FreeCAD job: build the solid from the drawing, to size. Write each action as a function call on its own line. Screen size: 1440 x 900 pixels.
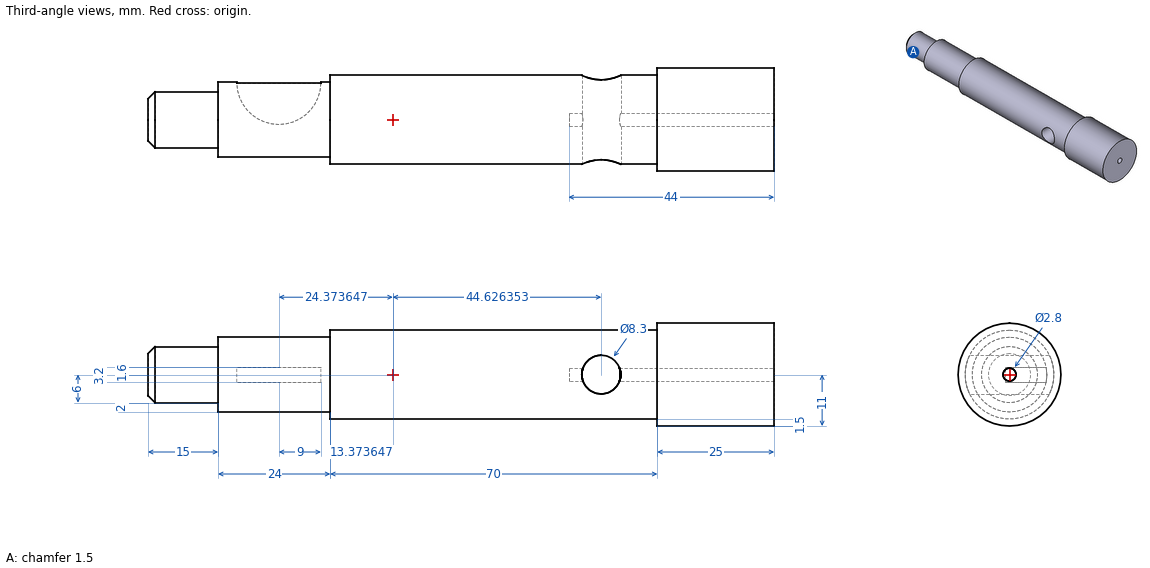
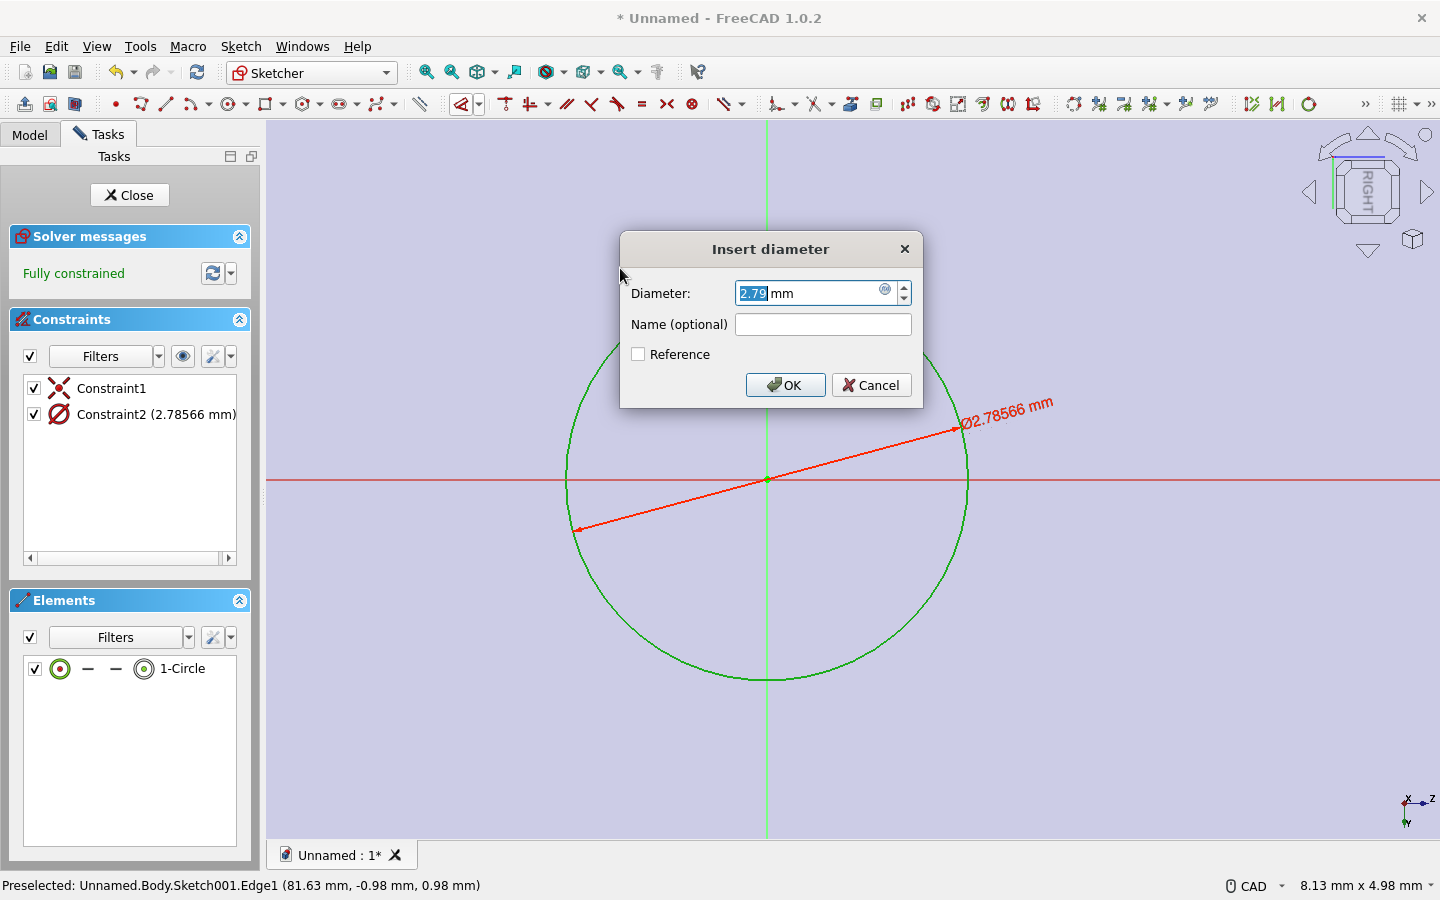
text(2.8)
key(Return)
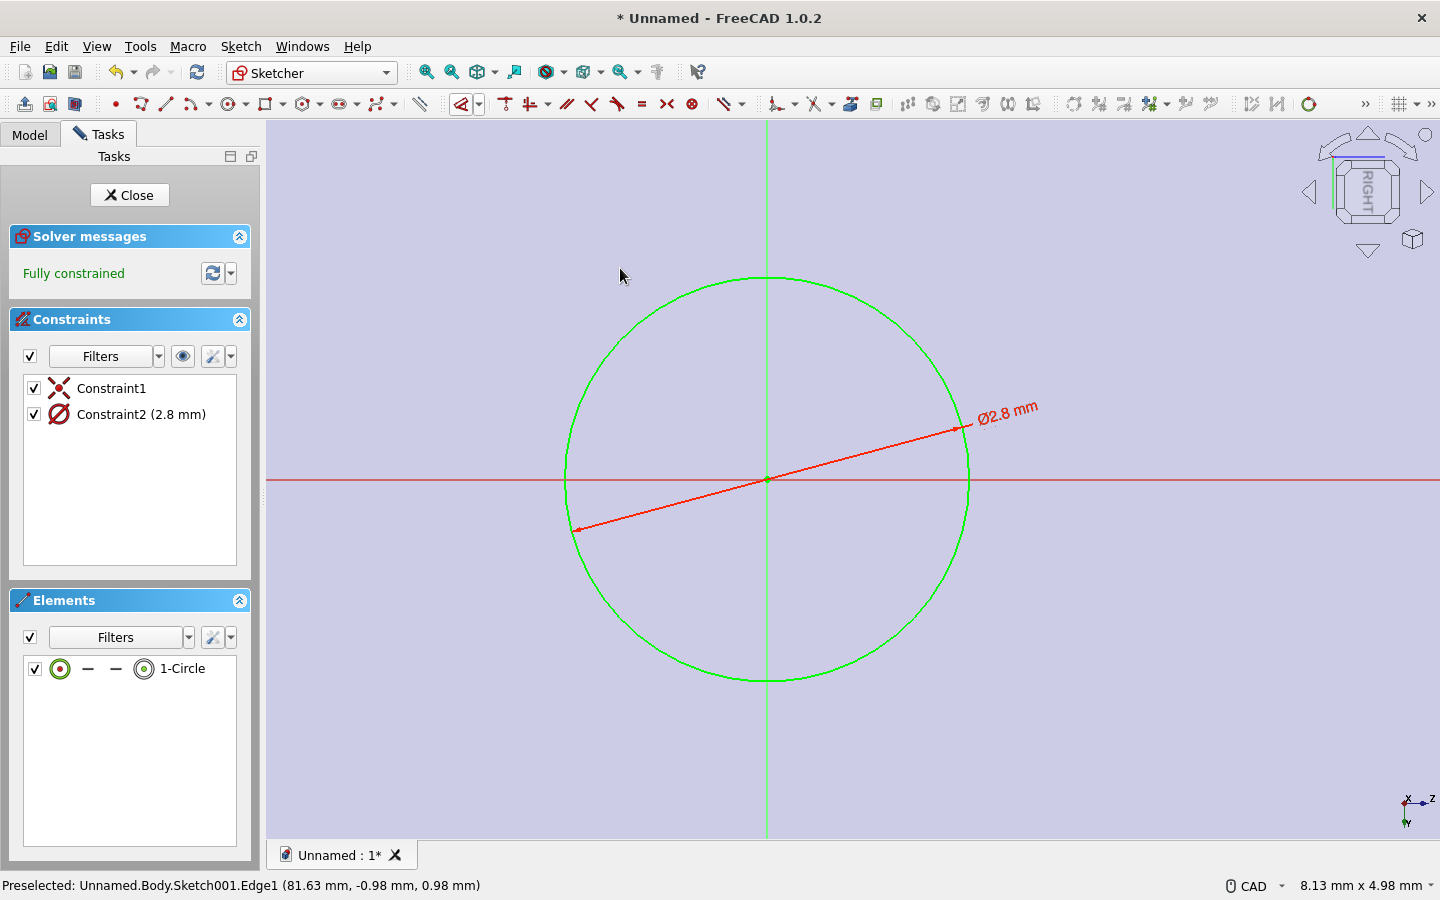
click(130, 195)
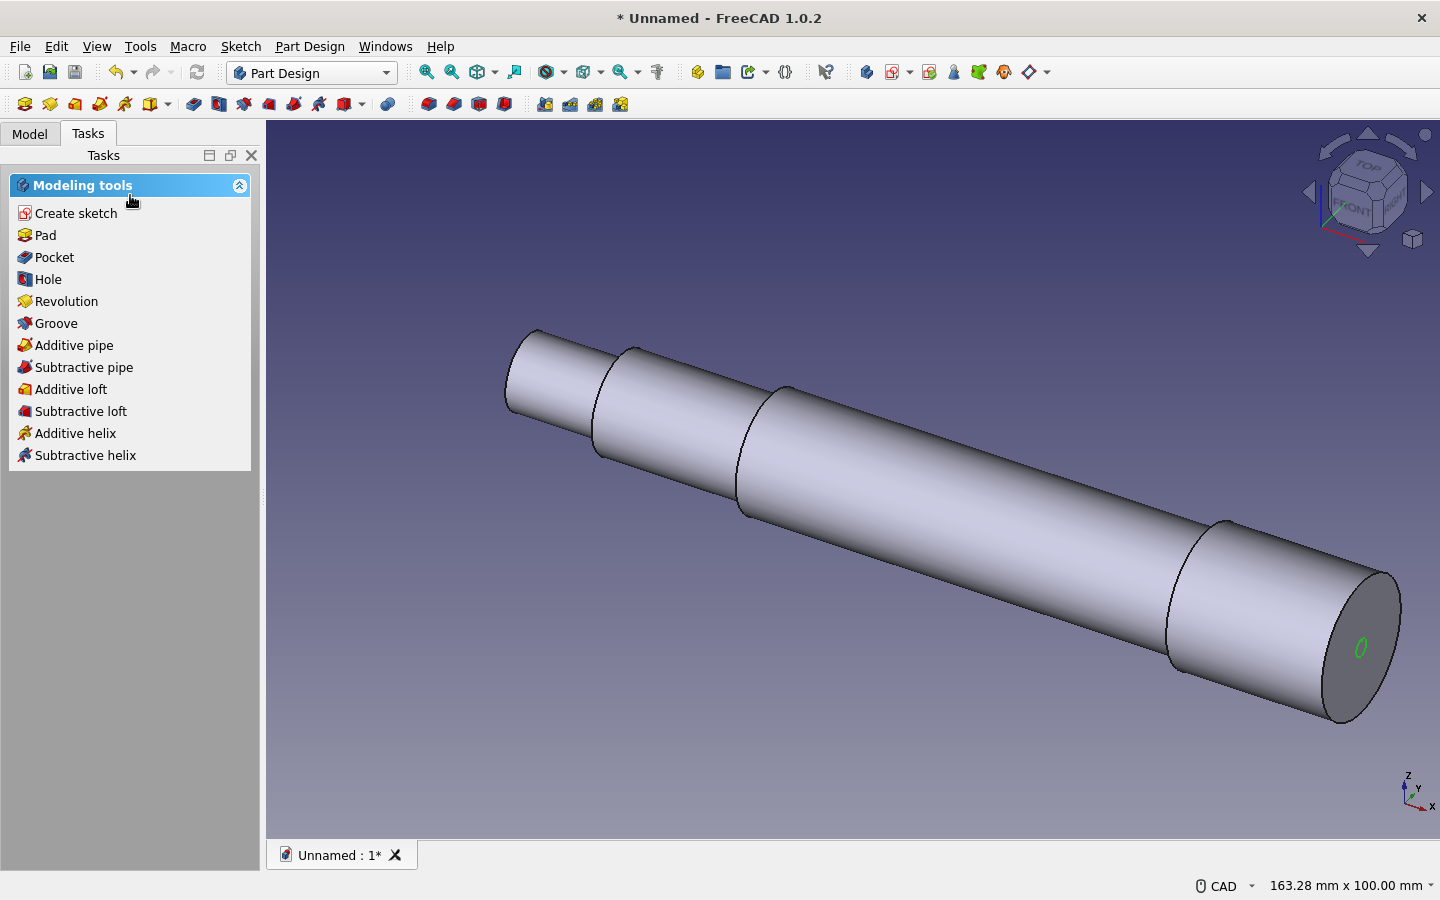
click(194, 104)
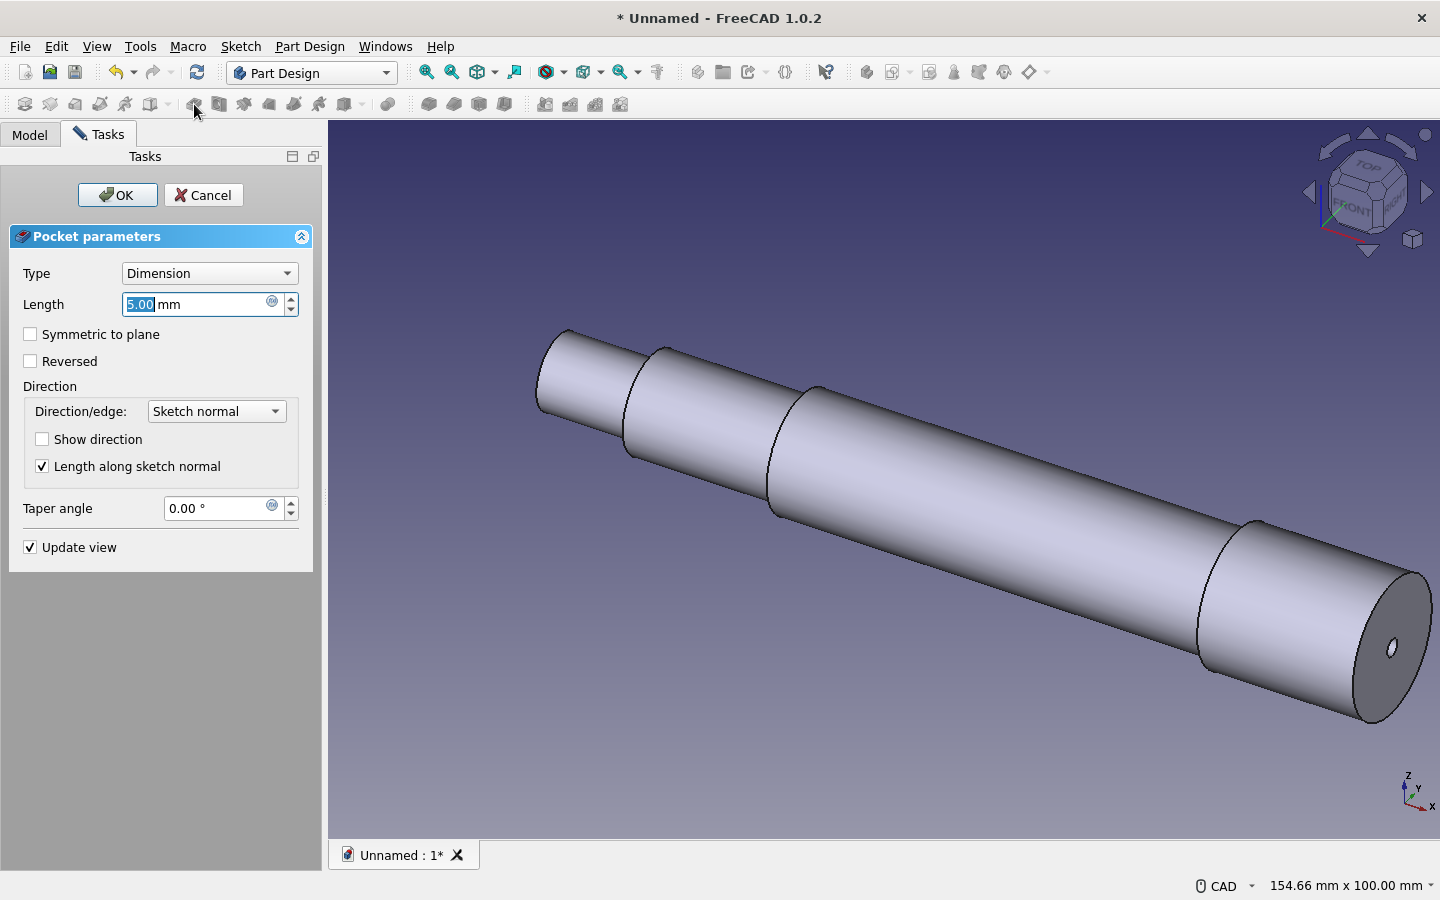
text(44)
key(Tab)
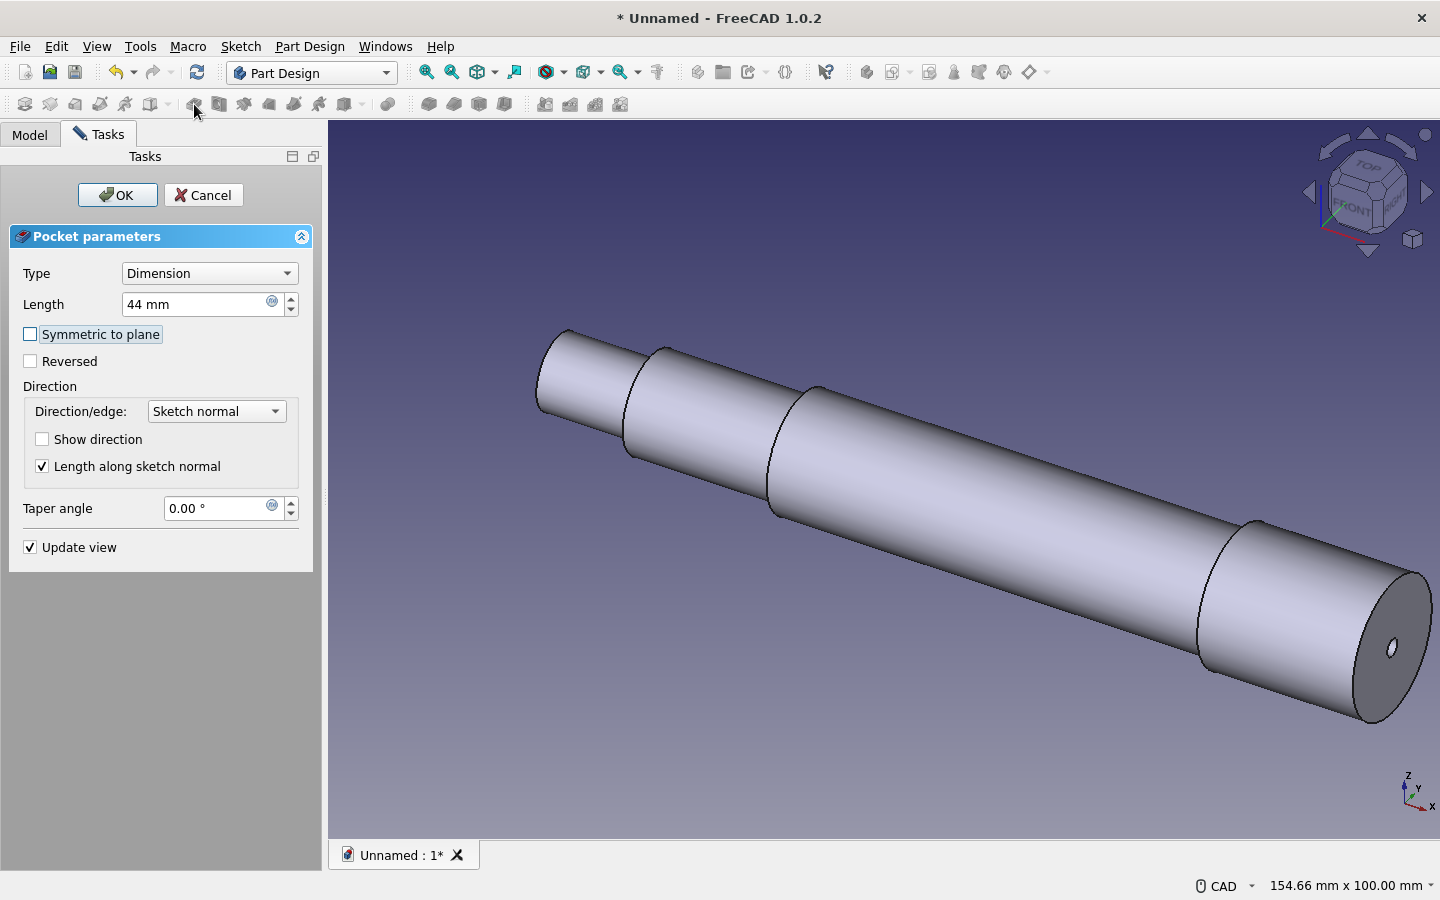
click(118, 195)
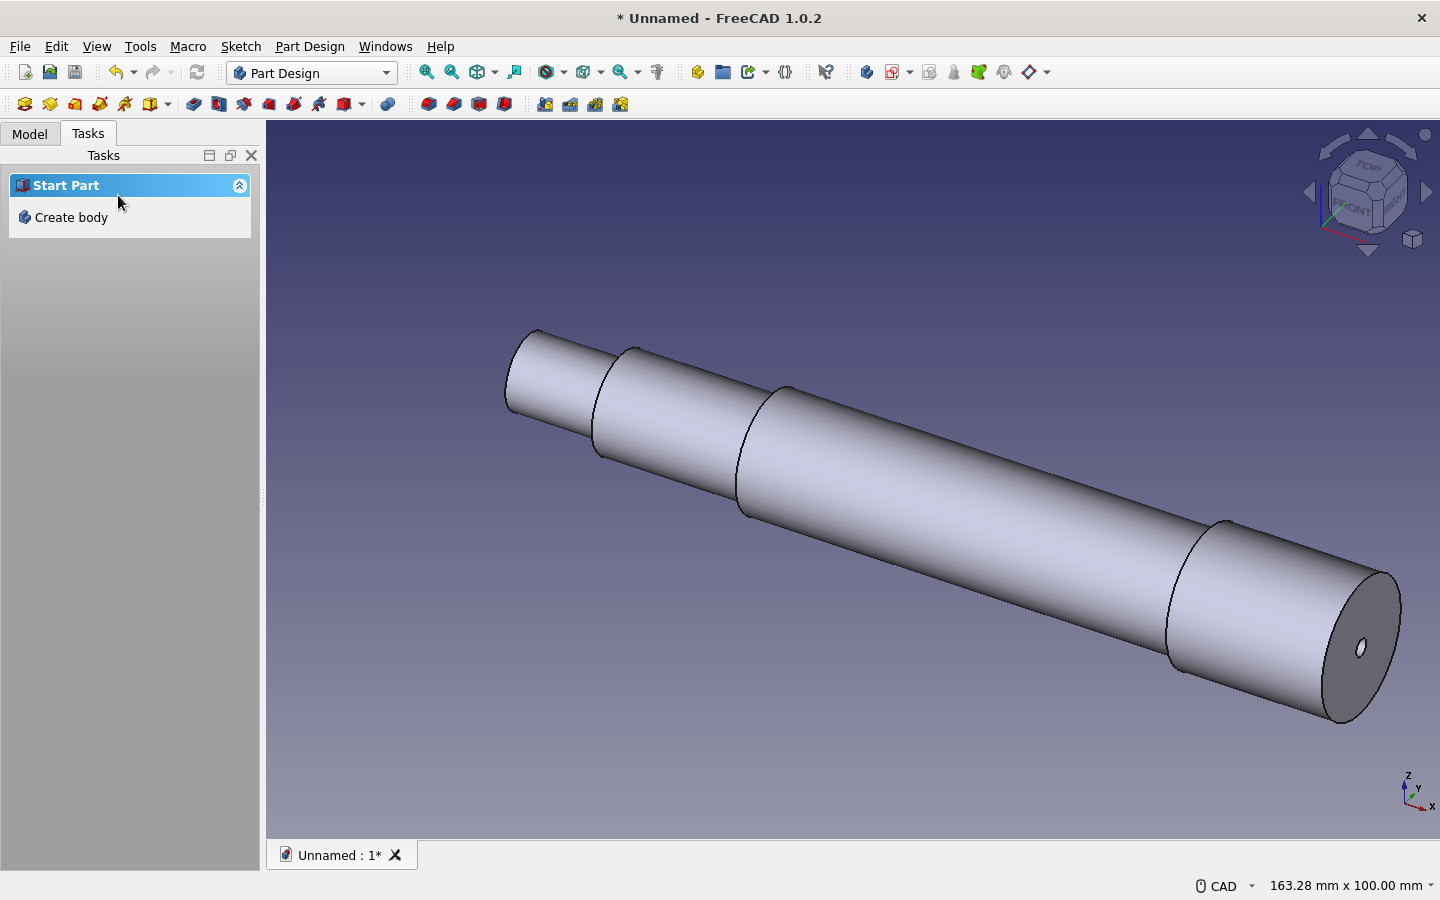
click(892, 72)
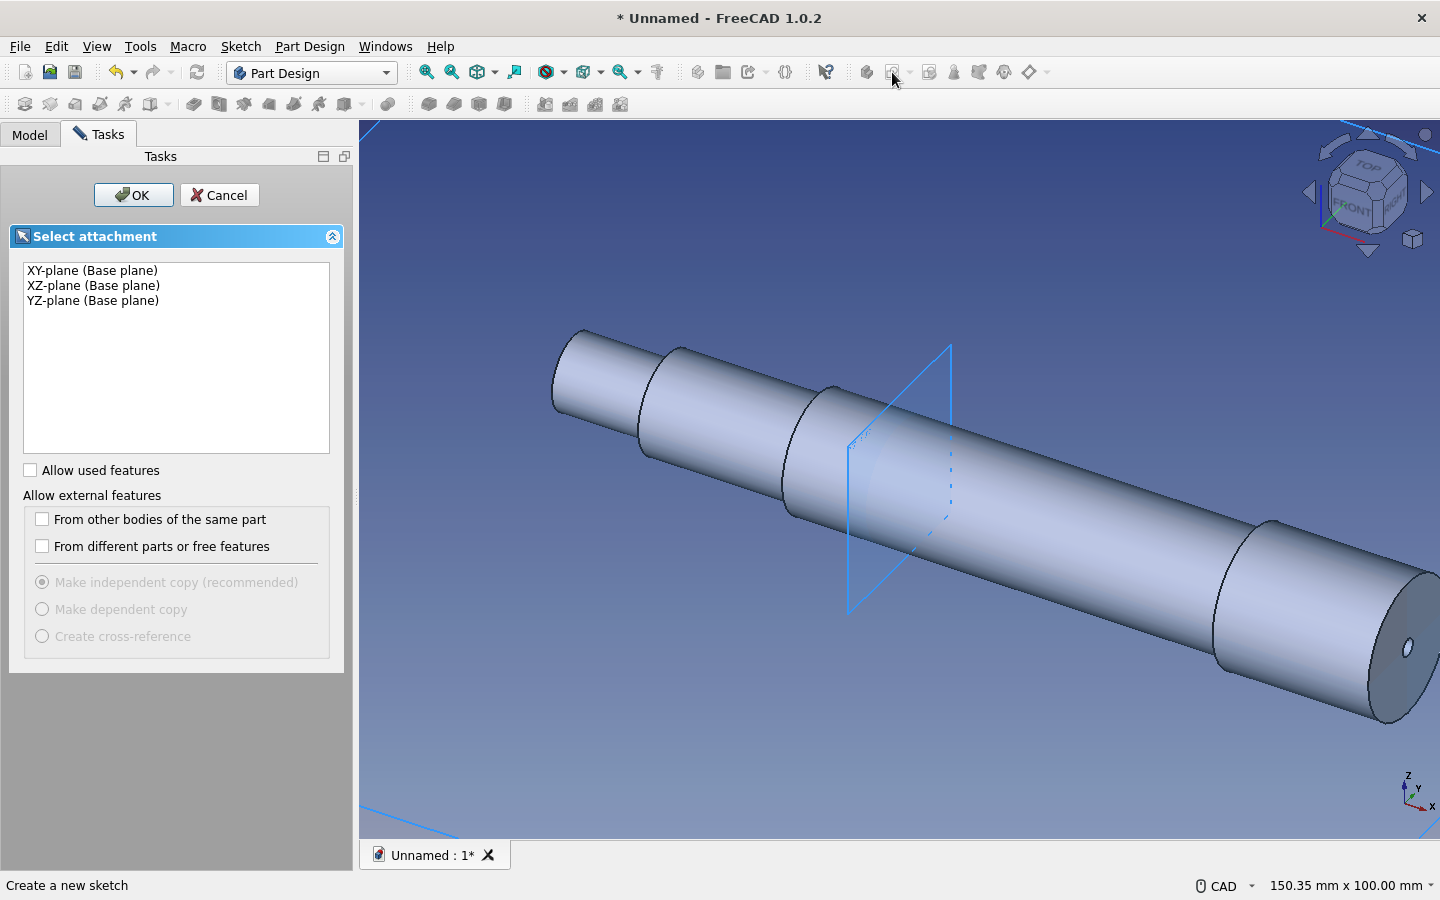
click(84, 286)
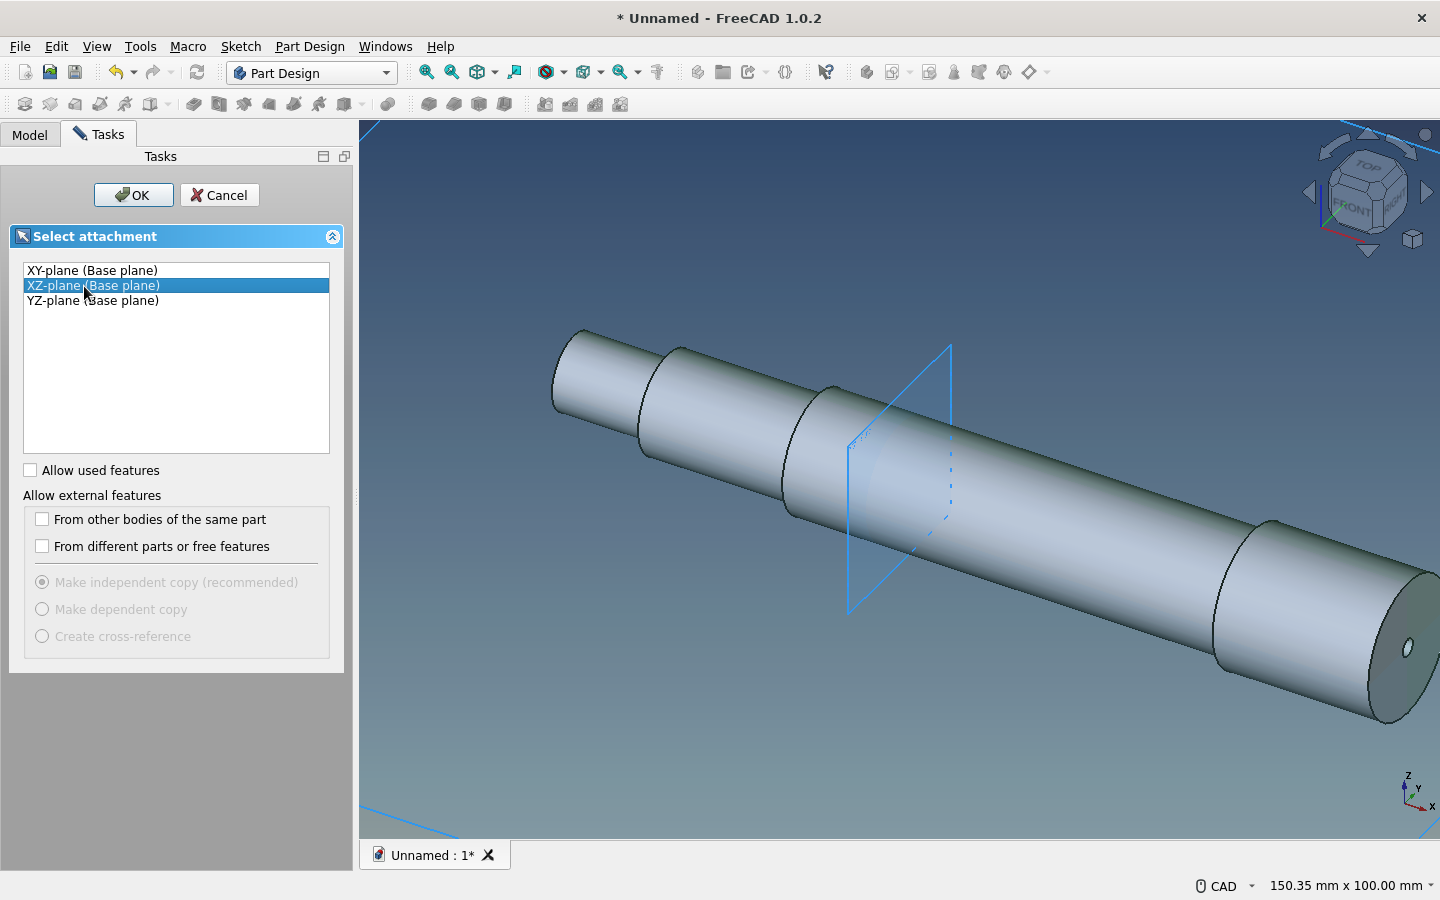
click(134, 195)